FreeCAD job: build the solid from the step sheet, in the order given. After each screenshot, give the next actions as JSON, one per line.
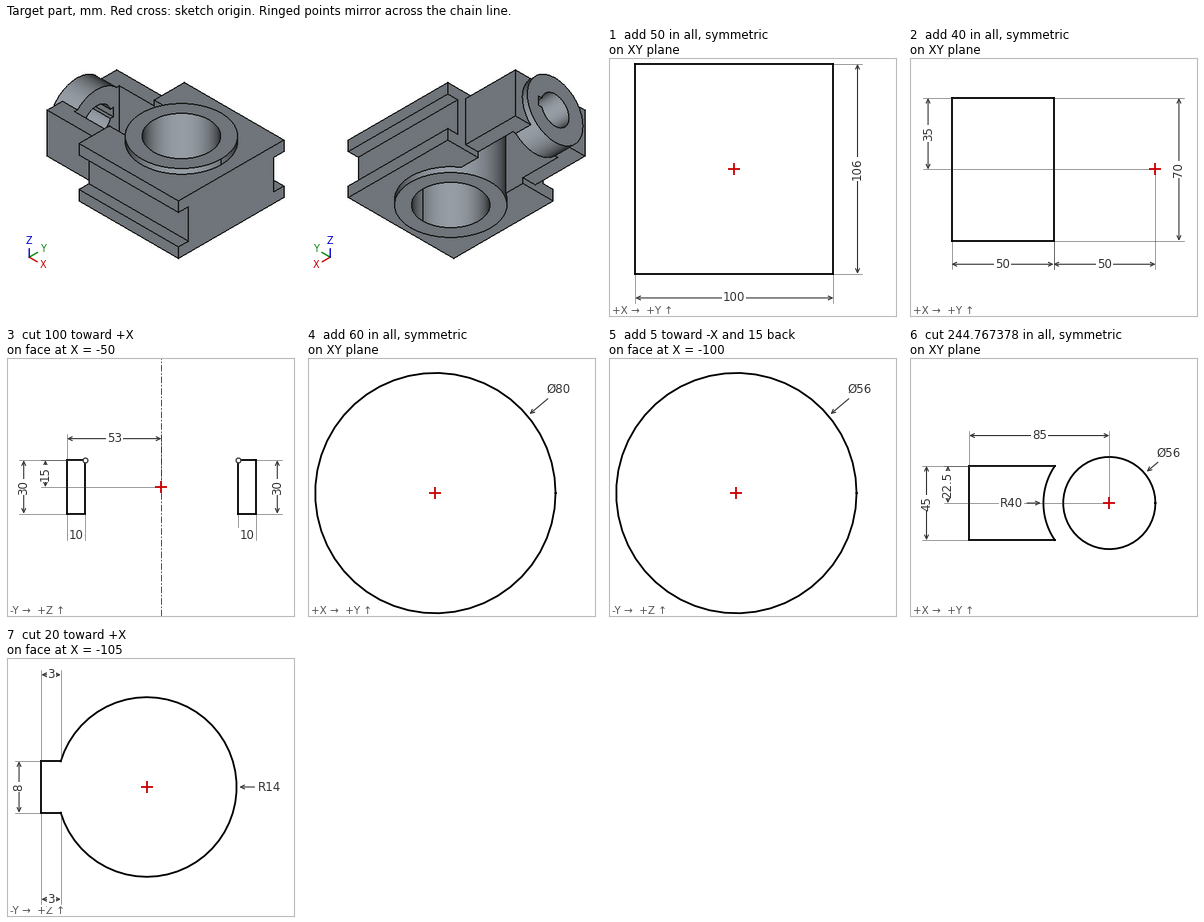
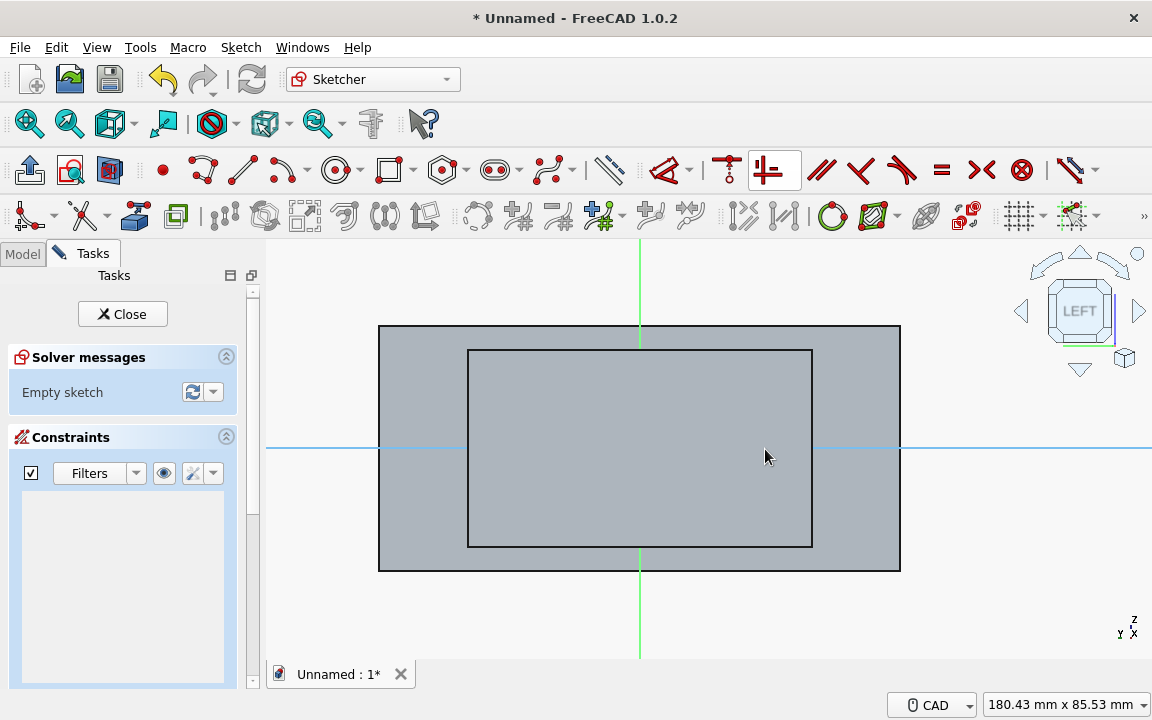
{"action": "left_click", "coordinate": [390, 170]}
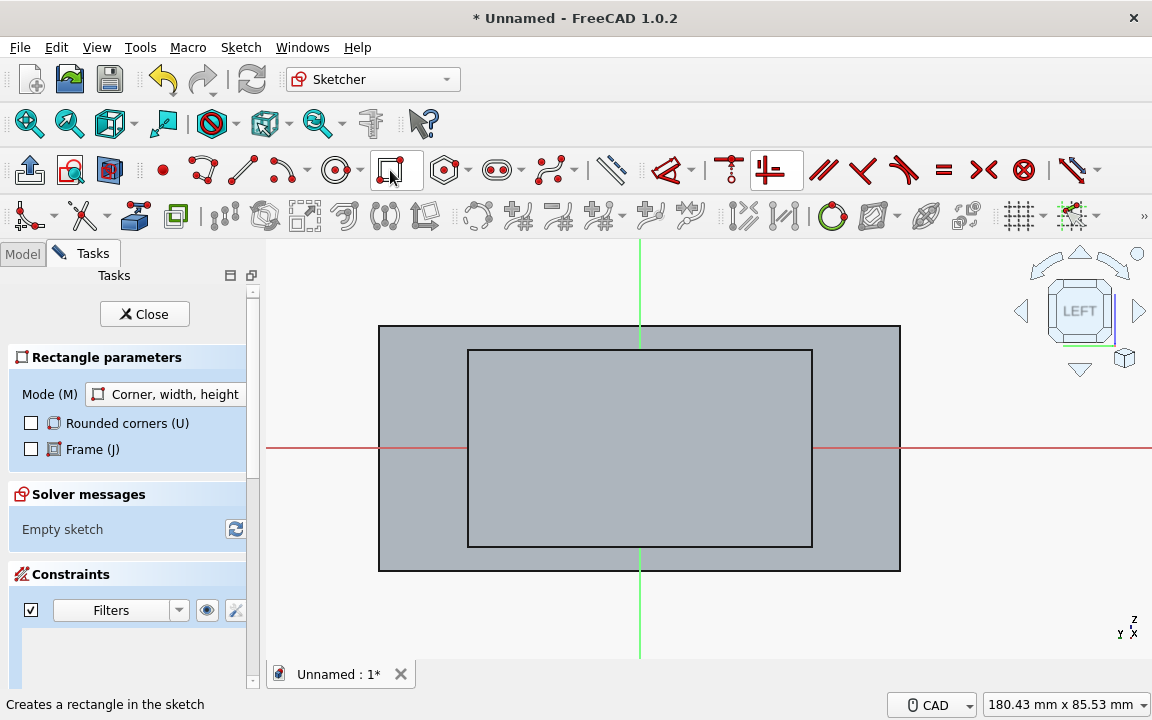
{"action": "left_click", "coordinate": [379, 375]}
{"action": "mouse_move", "coordinate": [429, 522]}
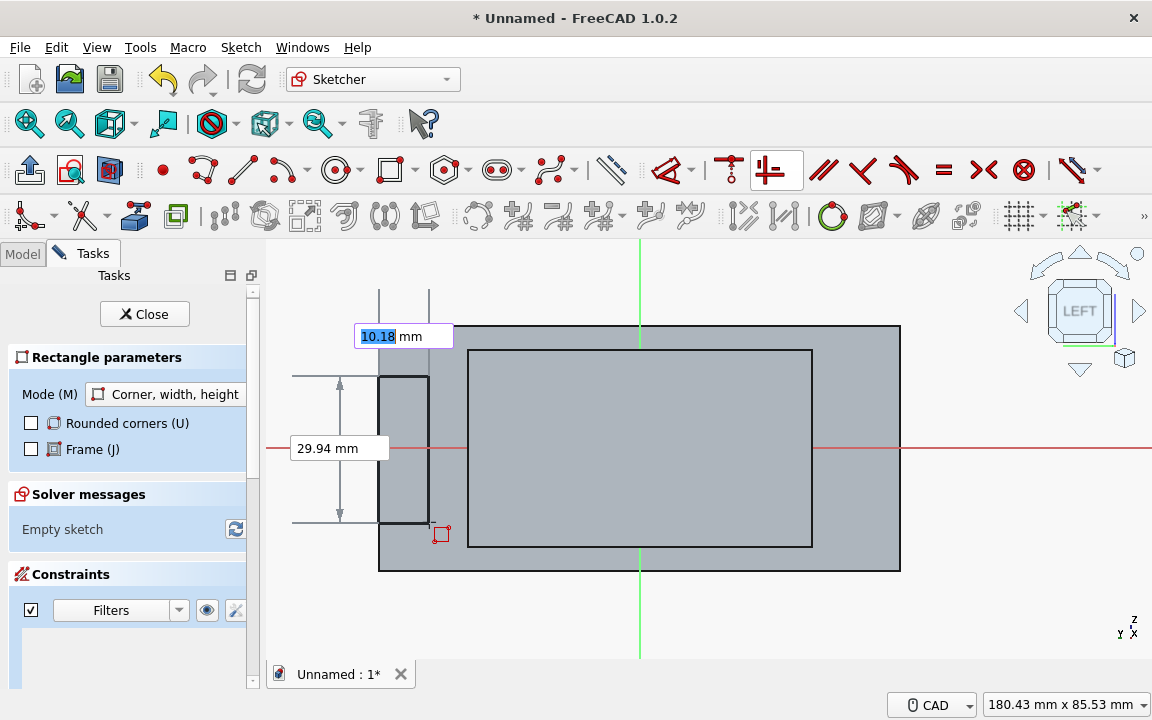
{"action": "type", "text": "10"}
{"action": "key", "text": "Tab"}
{"action": "type", "text": "30"}
{"action": "key", "text": "Return"}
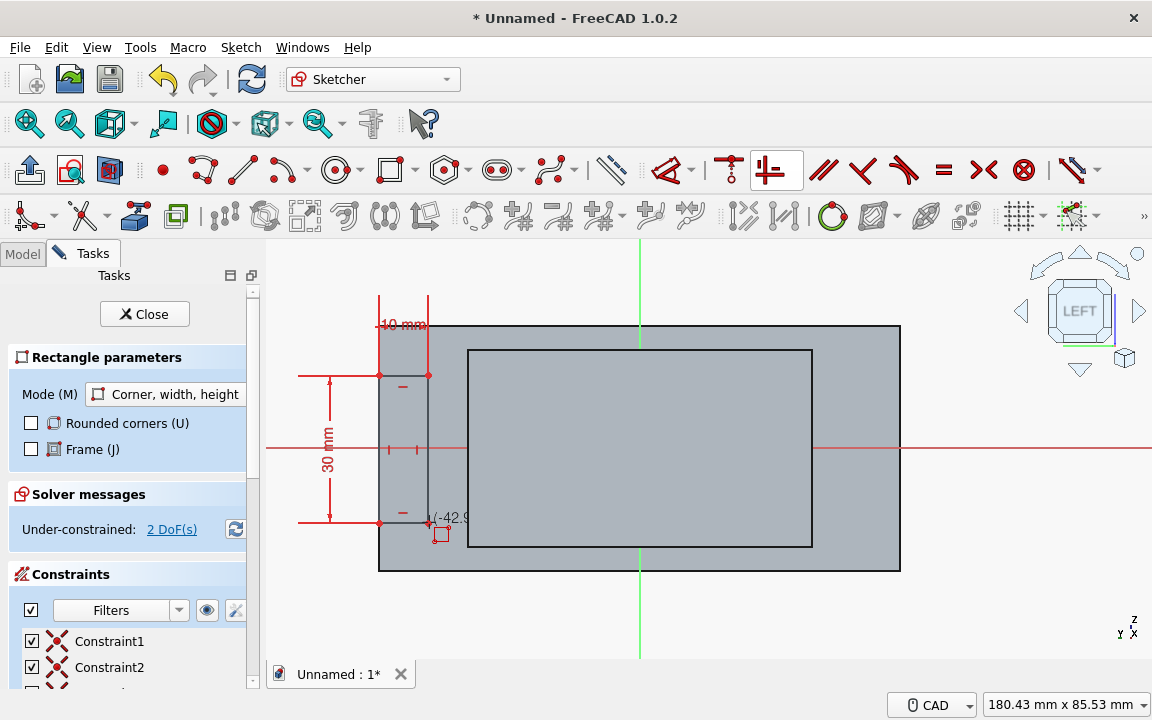
{"action": "left_click", "coordinate": [851, 375]}
{"action": "mouse_move", "coordinate": [900, 522]}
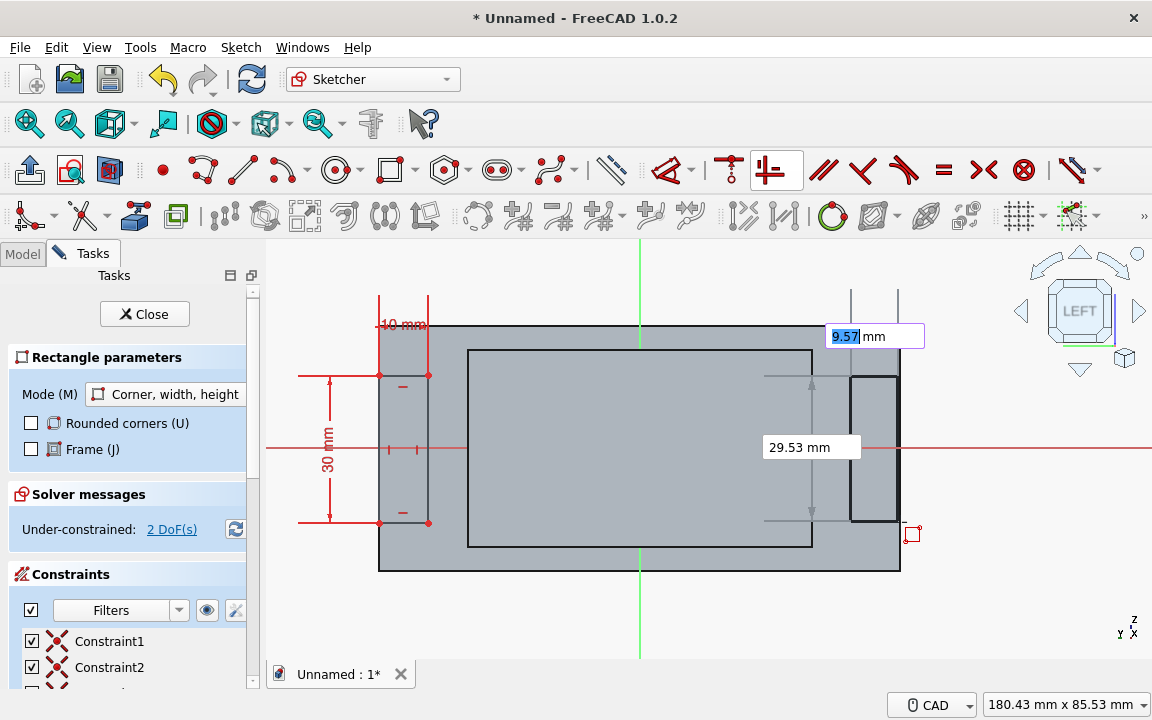
{"action": "type", "text": "10"}
{"action": "key", "text": "Tab"}
{"action": "type", "text": "30"}
{"action": "key", "text": "Return"}
{"action": "key", "text": "Escape"}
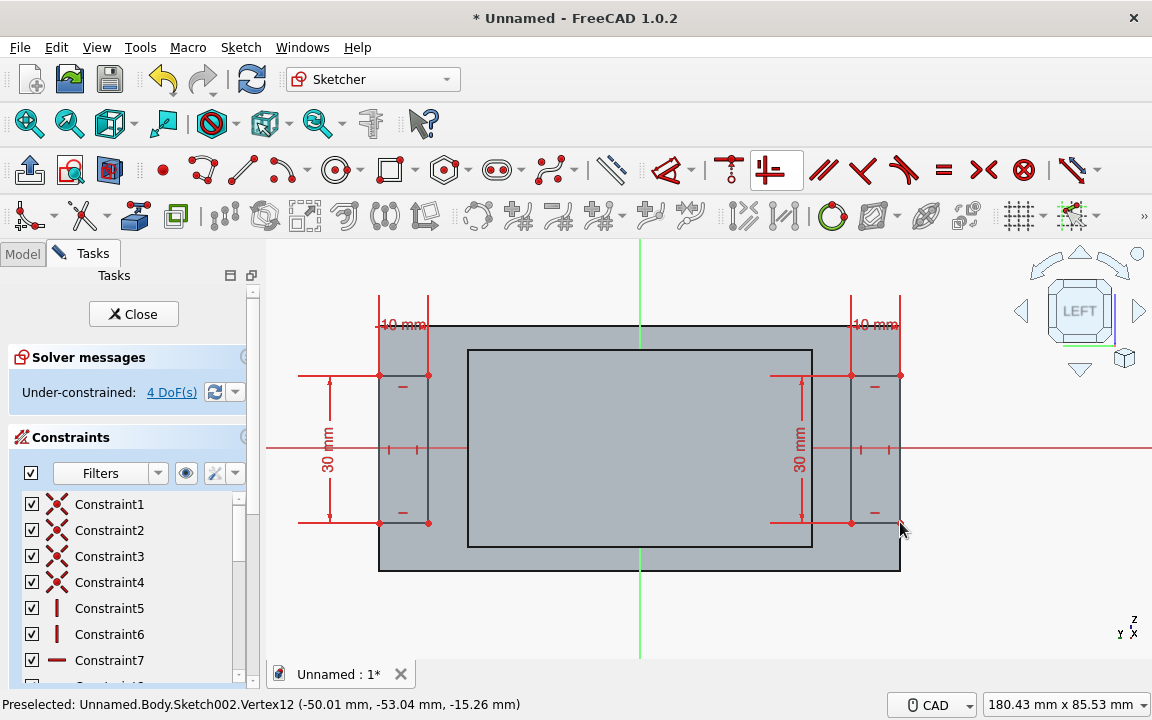
{"action": "left_click", "coordinate": [428, 376]}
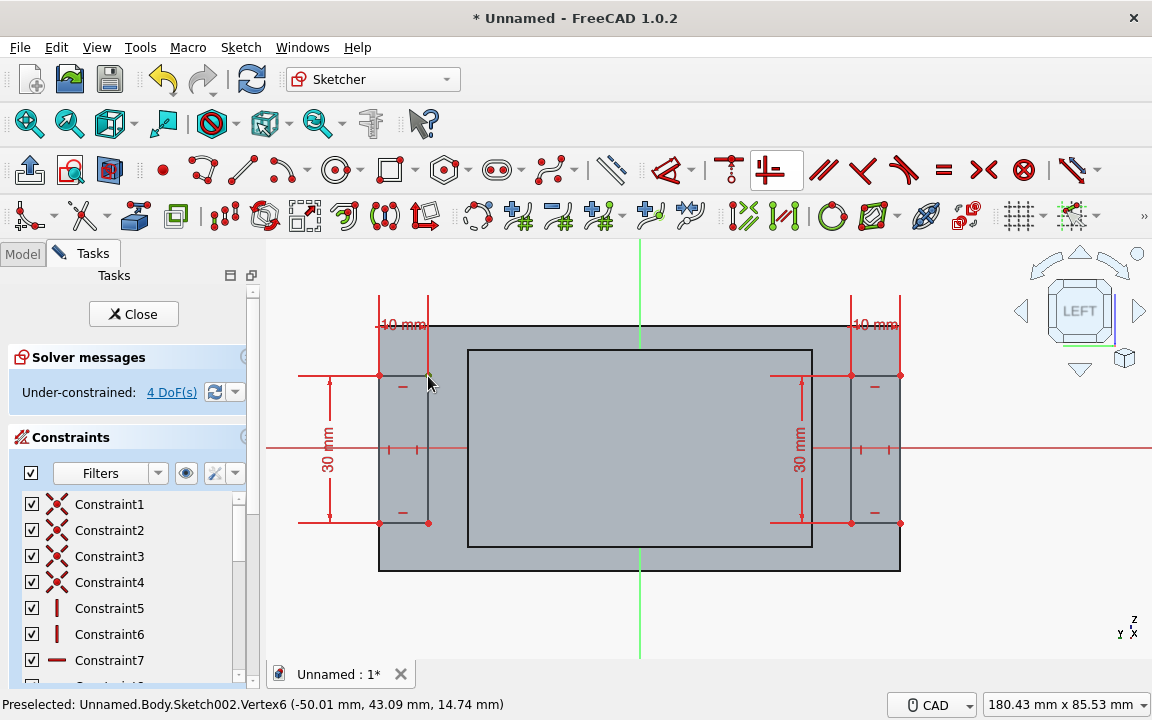
{"action": "left_click", "coordinate": [851, 376]}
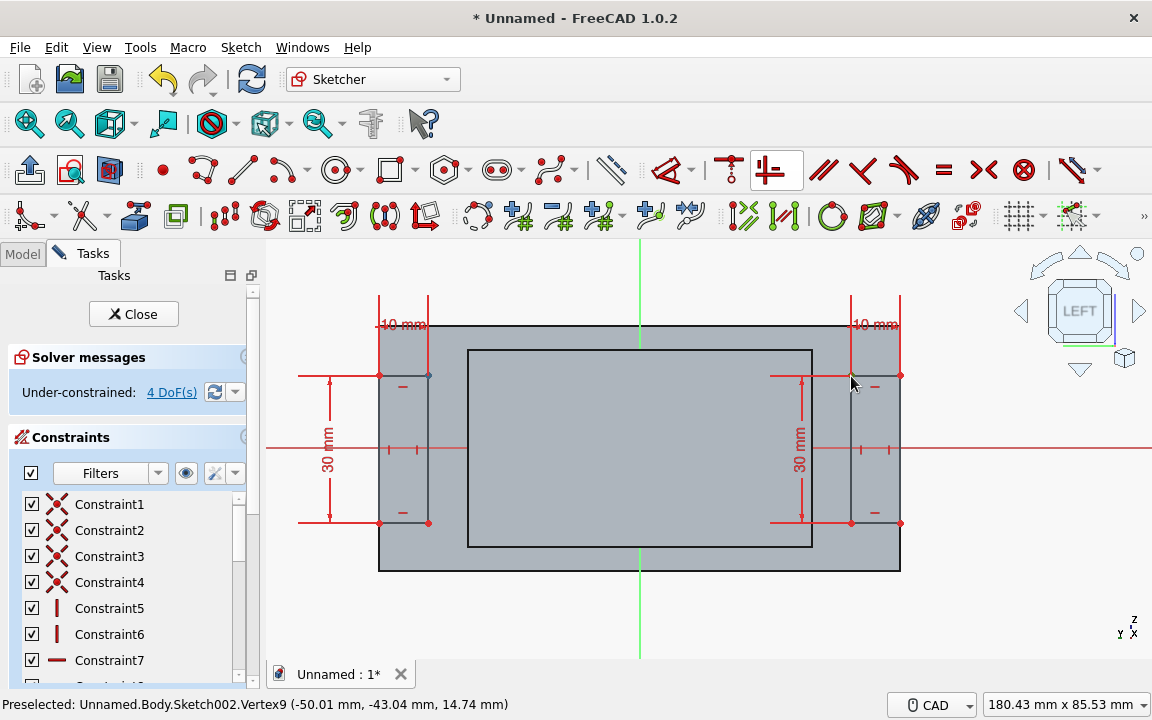
{"action": "left_click", "coordinate": [640, 605]}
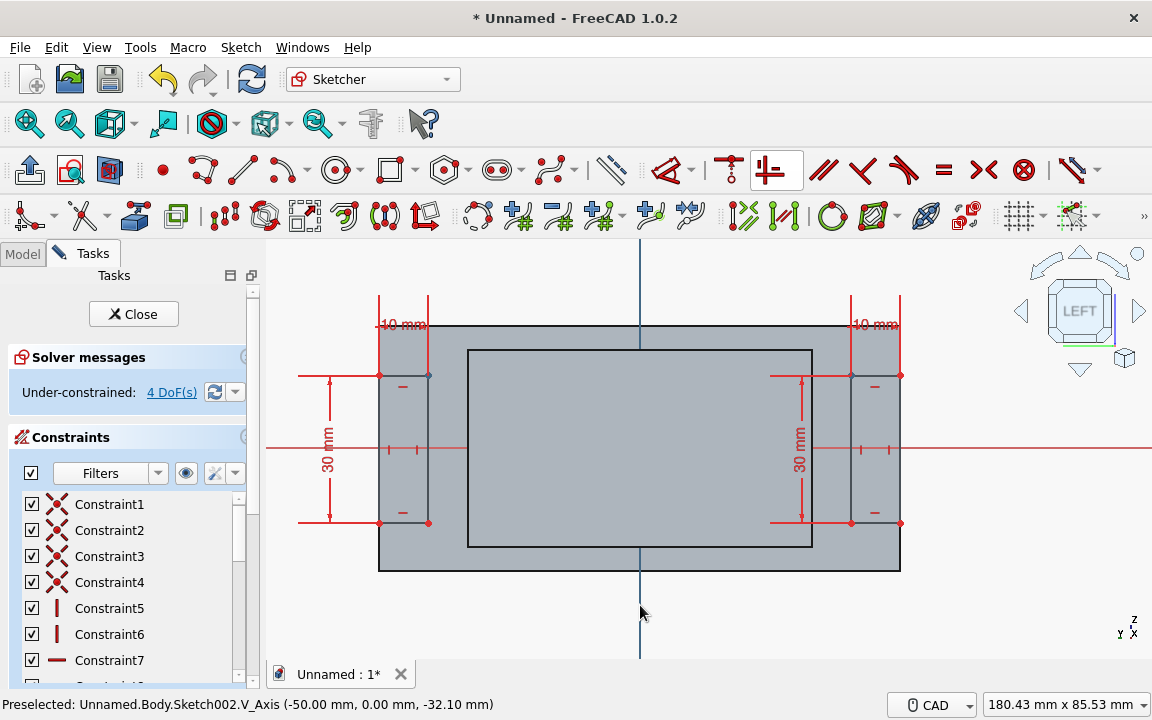
{"action": "left_click", "coordinate": [984, 170]}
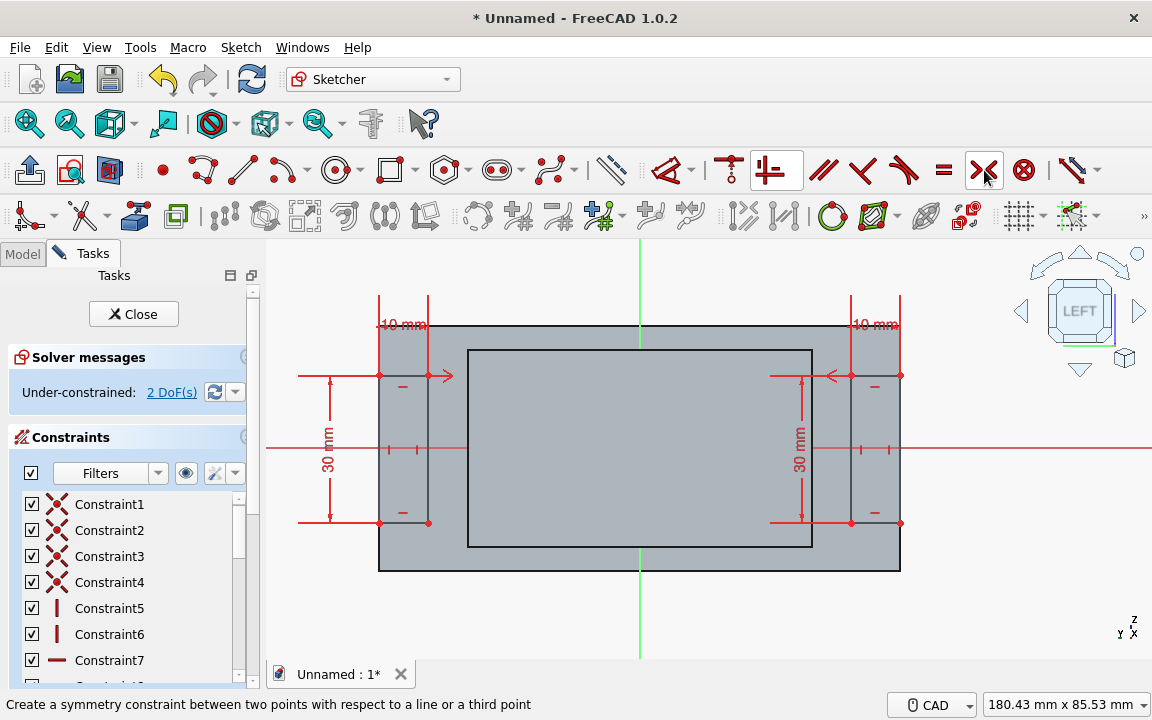
{"action": "left_click", "coordinate": [666, 170]}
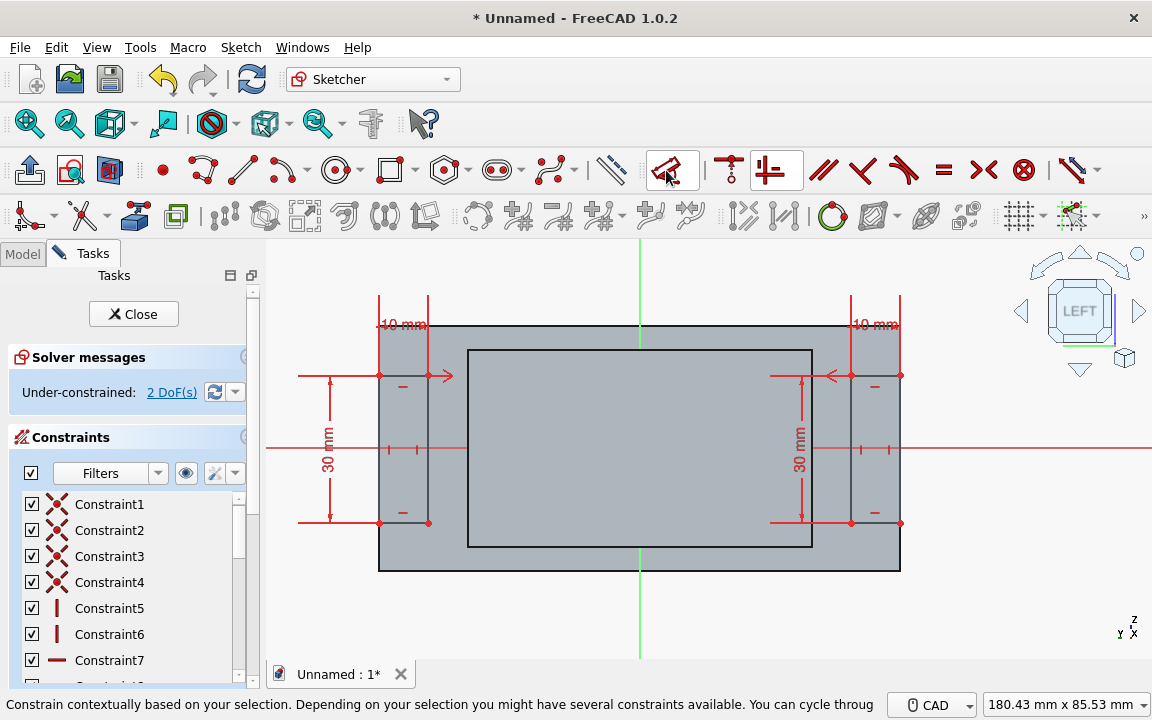
{"action": "left_click", "coordinate": [379, 376]}
{"action": "left_click", "coordinate": [509, 342]}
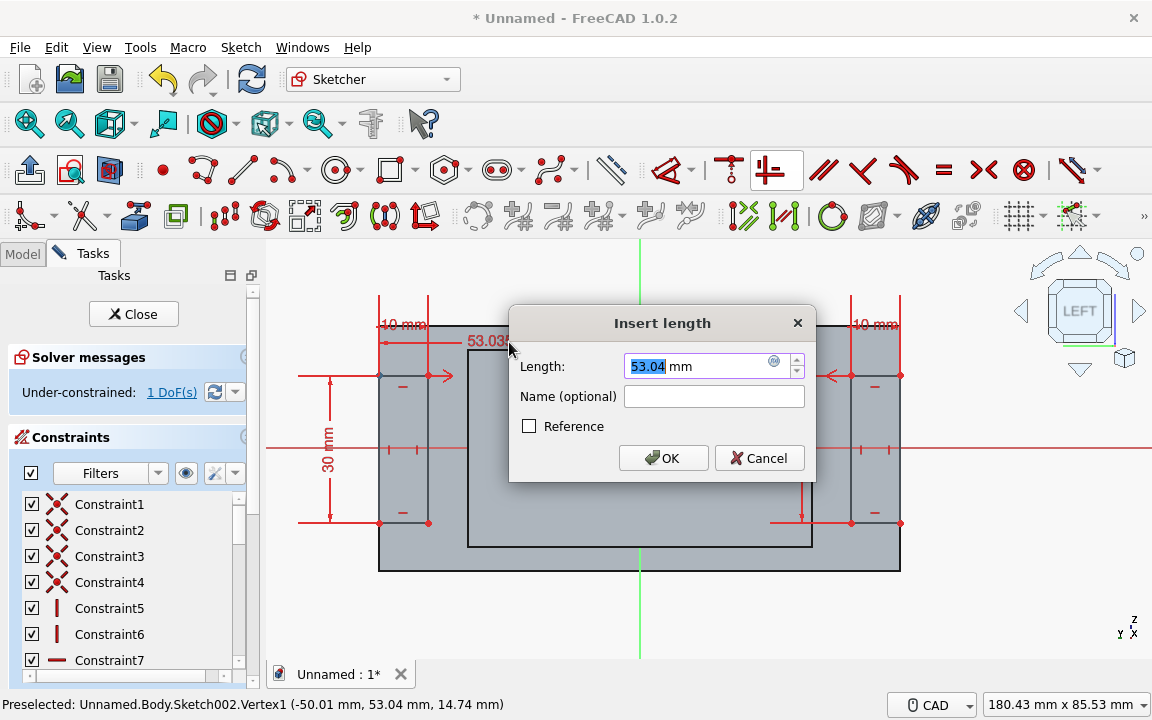
{"action": "type", "text": "53"}
{"action": "key", "text": "Return"}